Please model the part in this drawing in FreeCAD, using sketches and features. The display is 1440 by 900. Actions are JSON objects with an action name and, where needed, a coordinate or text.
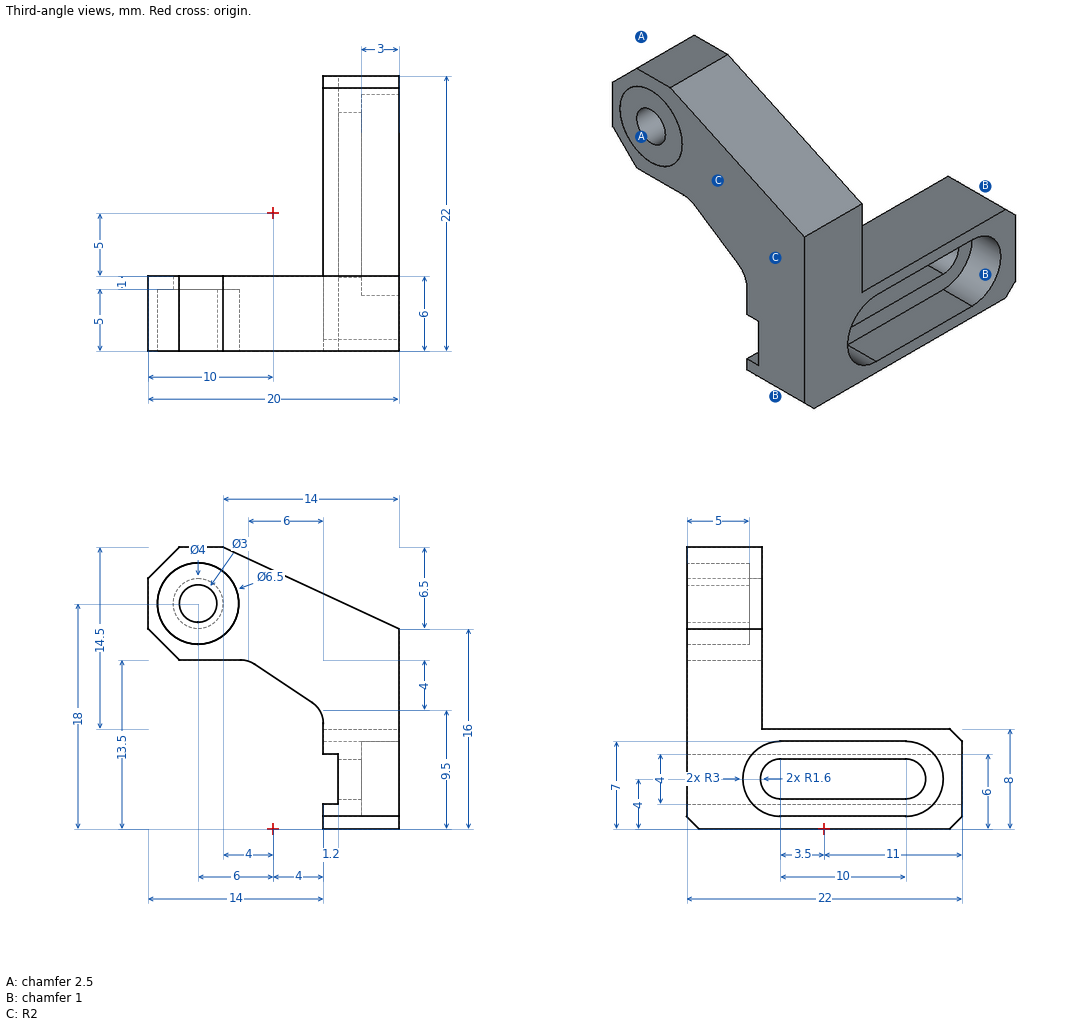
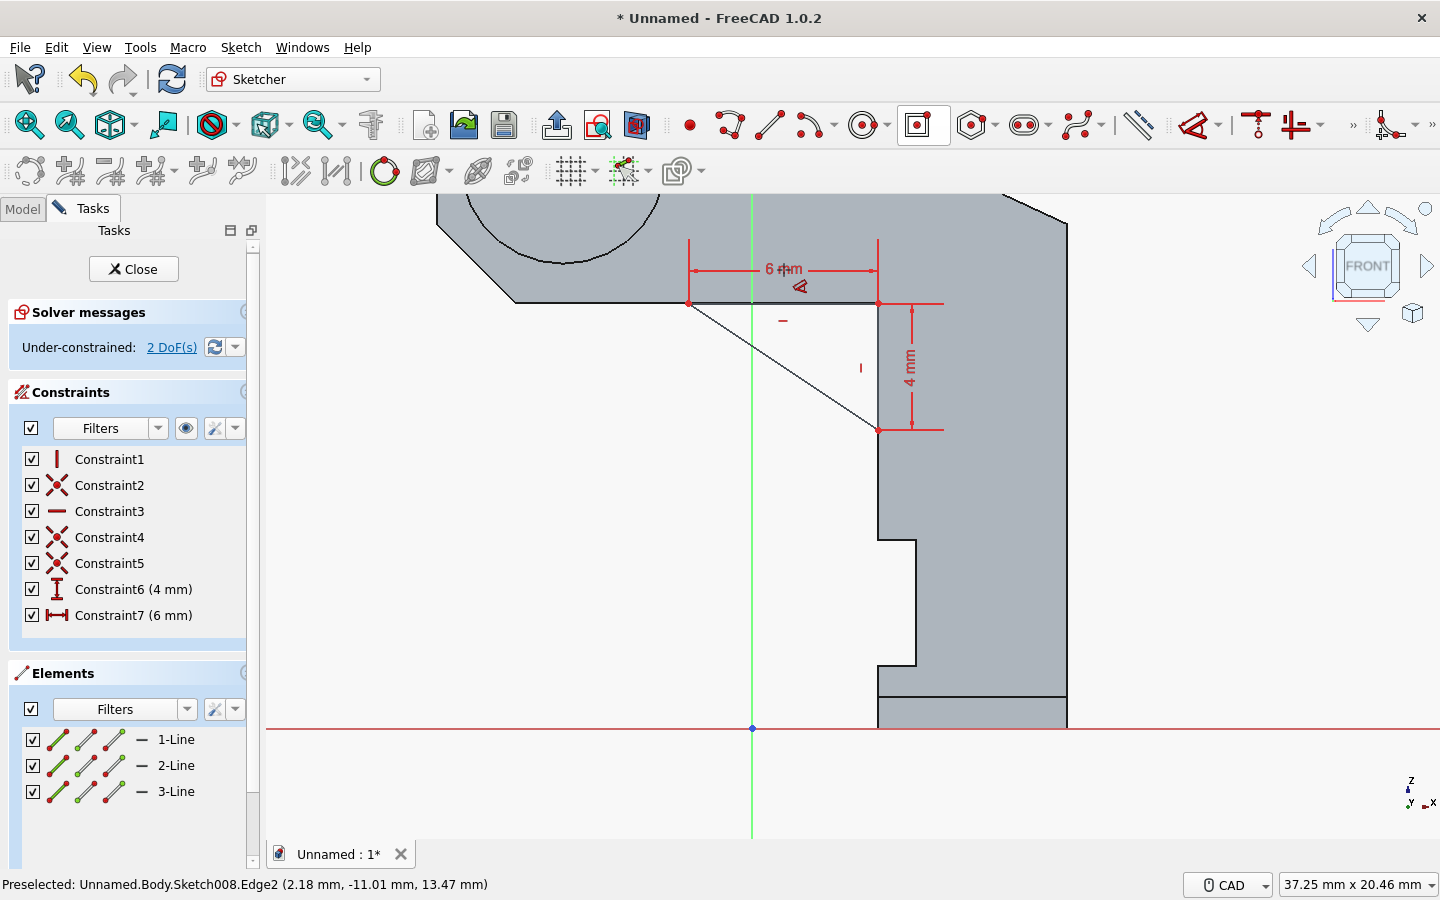
{"action": "left_click", "coordinate": [878, 430]}
{"action": "left_click", "coordinate": [815, 763]}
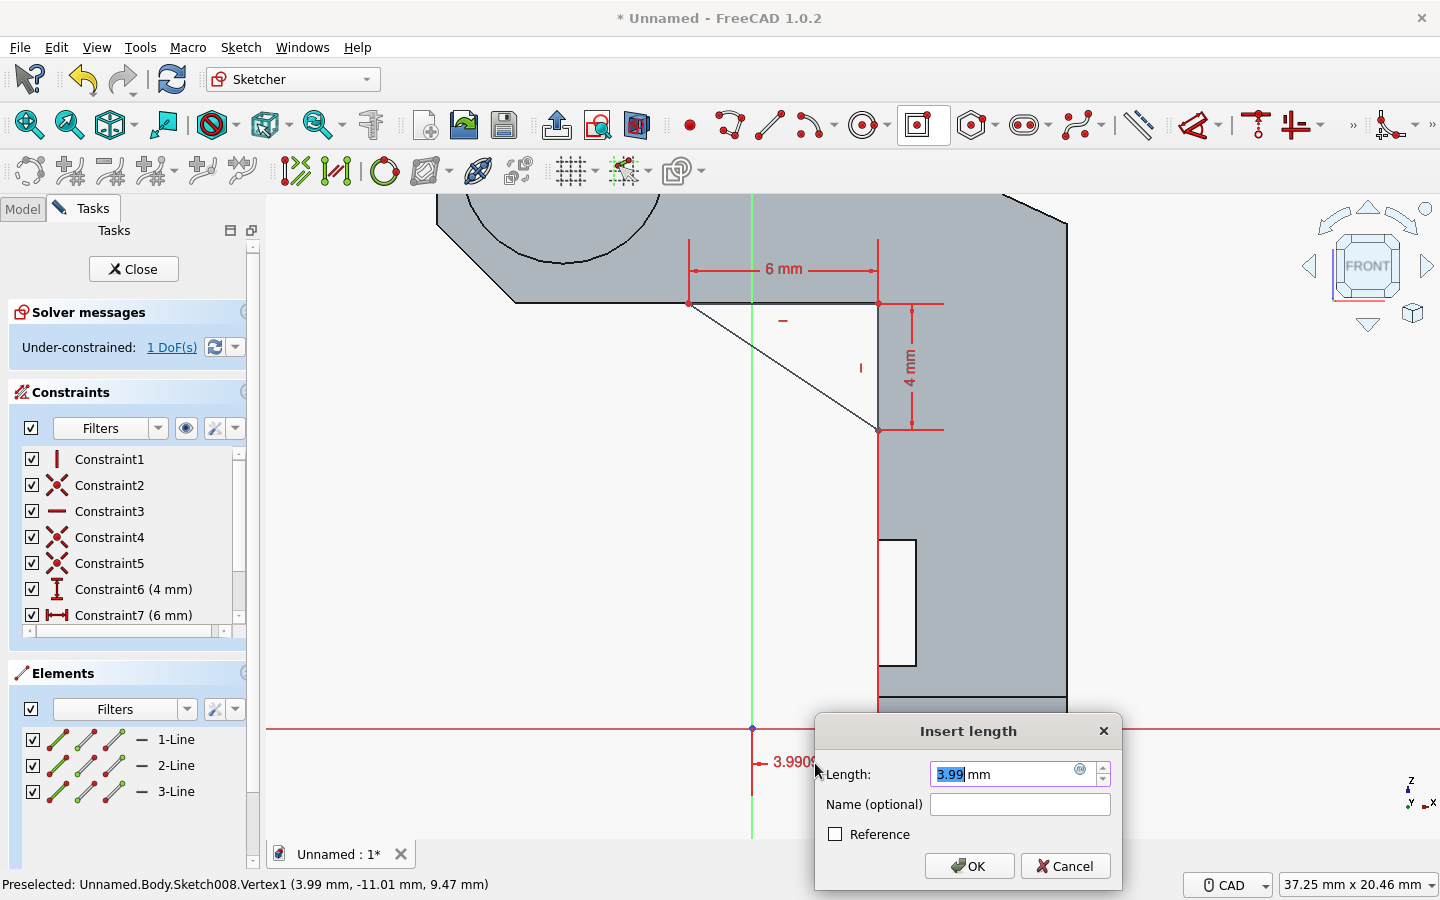
{"action": "type", "text": "4"}
{"action": "key", "text": "Return"}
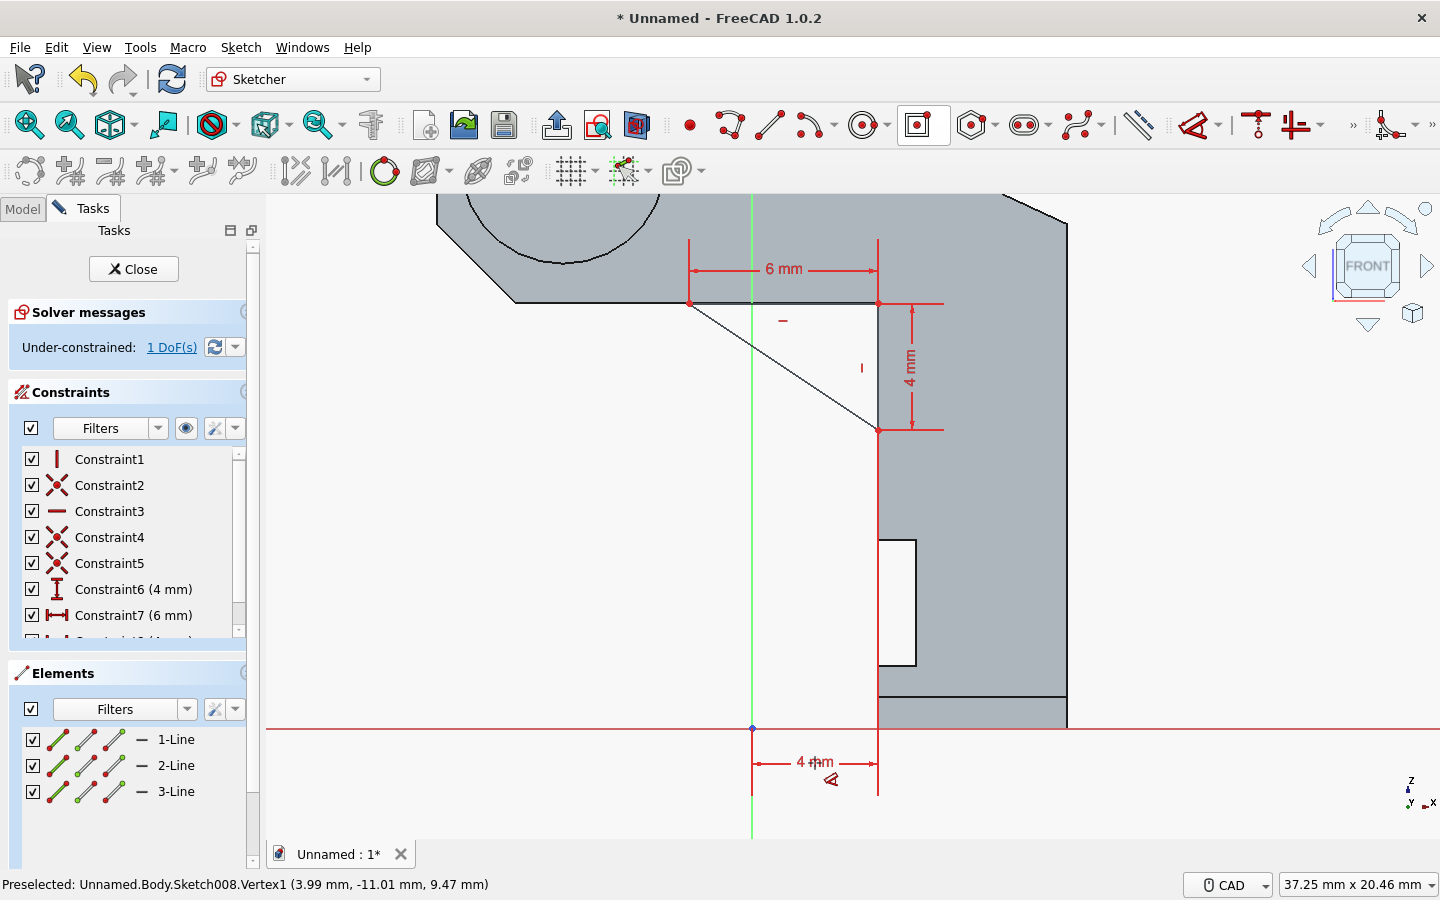
{"action": "left_click", "coordinate": [878, 430]}
{"action": "left_click", "coordinate": [912, 579]}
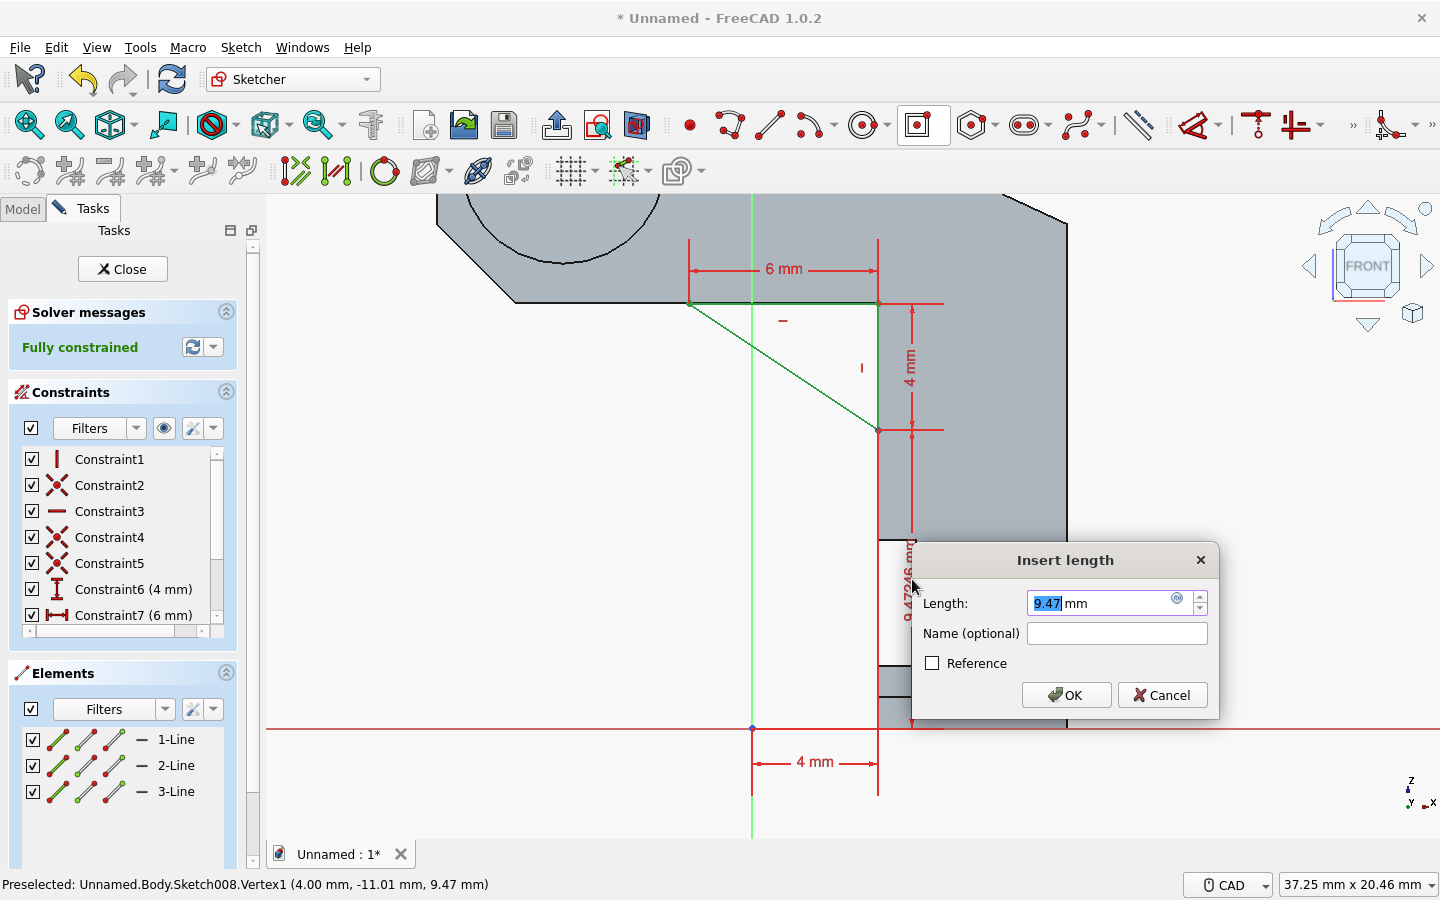
{"action": "type", "text": "9.5"}
{"action": "key", "text": "Return"}
{"action": "key", "text": "Escape"}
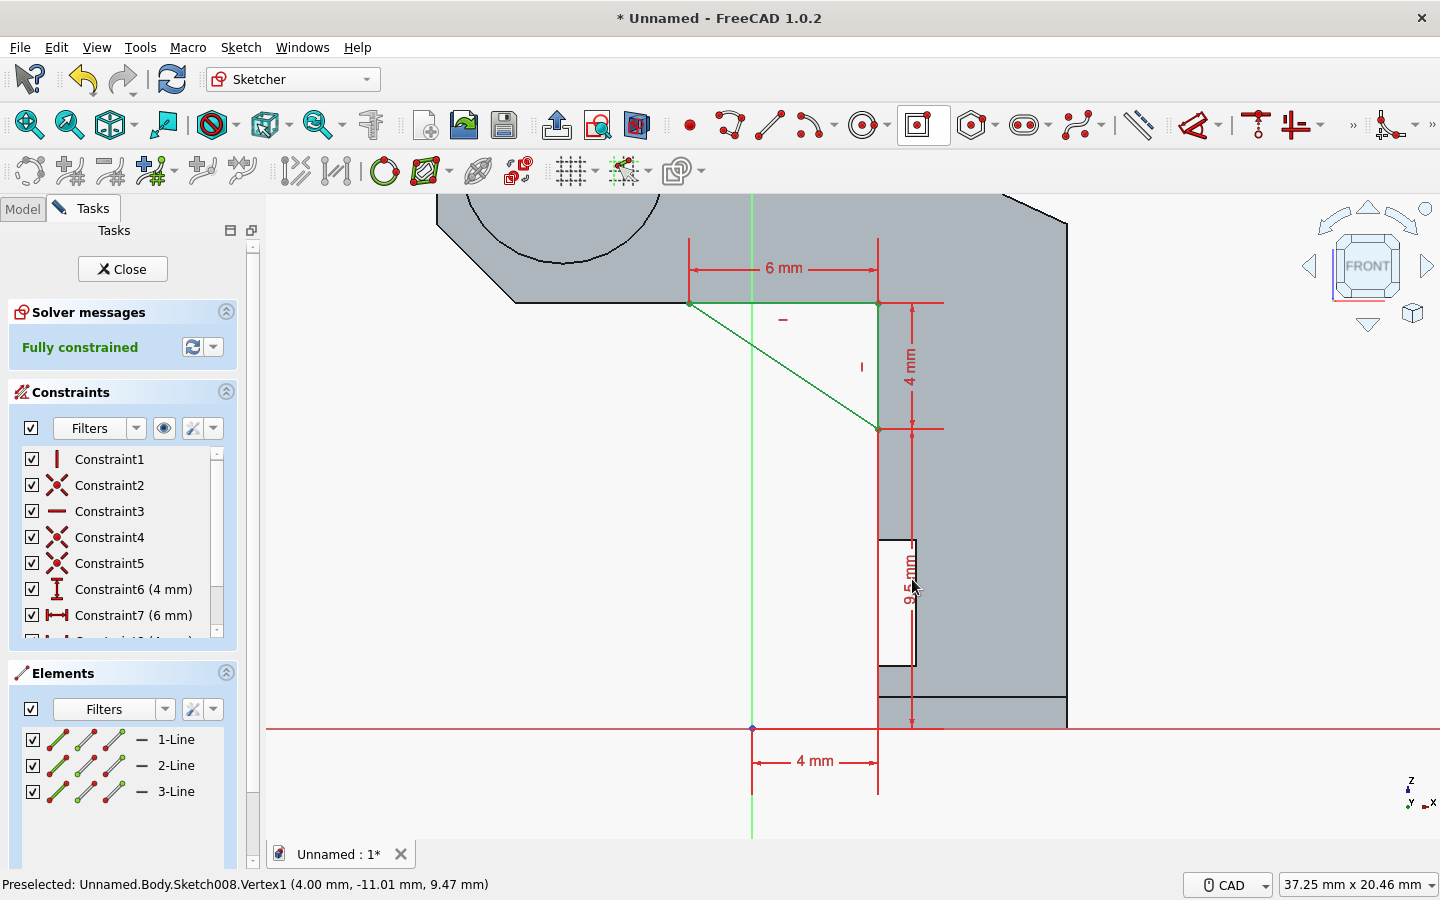
{"action": "left_click", "coordinate": [123, 269]}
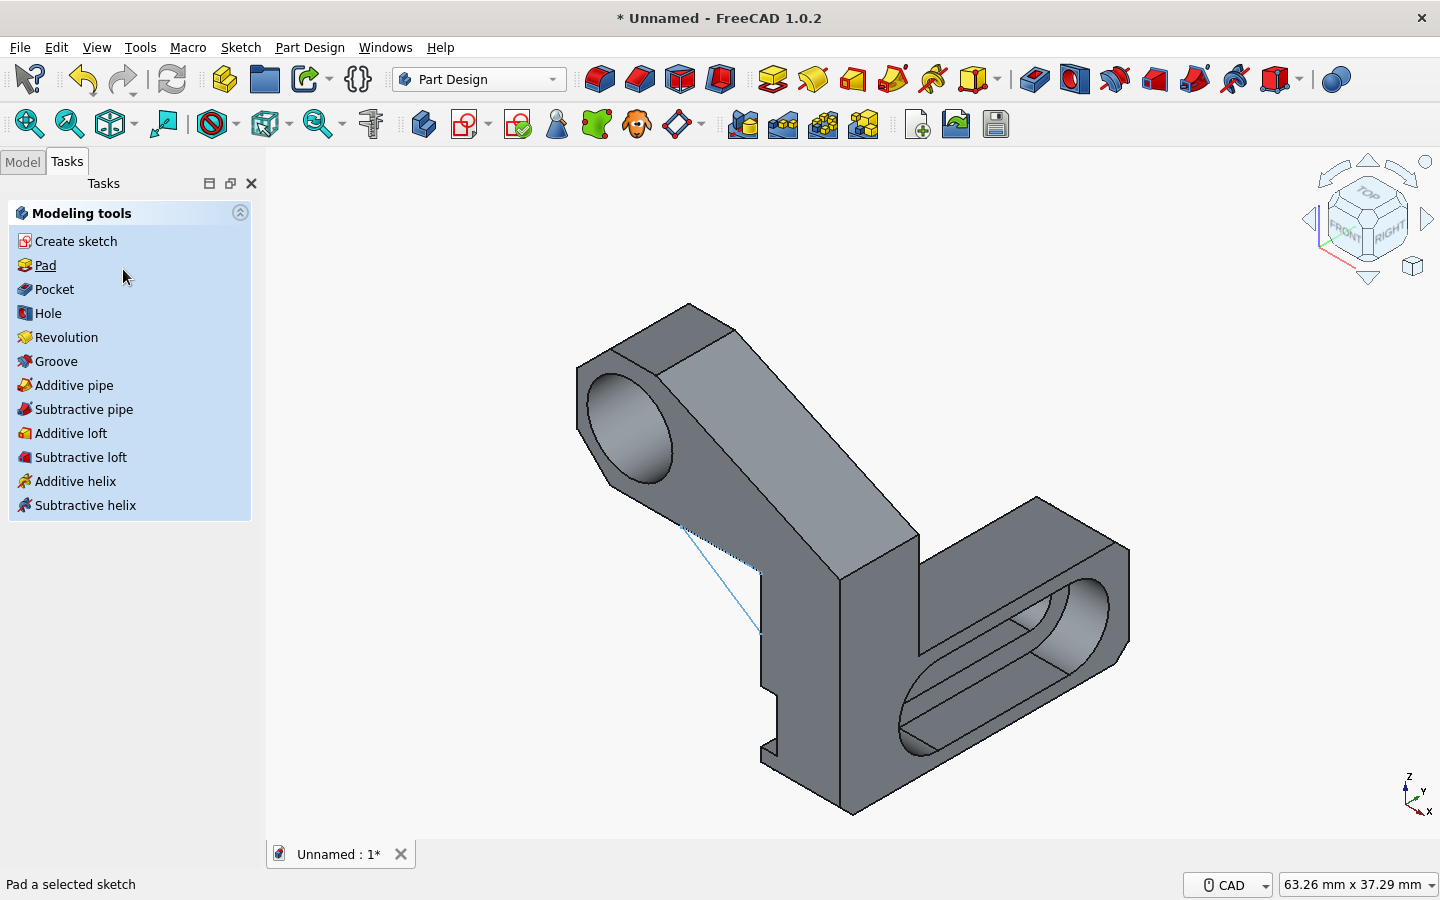
{"action": "left_click", "coordinate": [774, 80]}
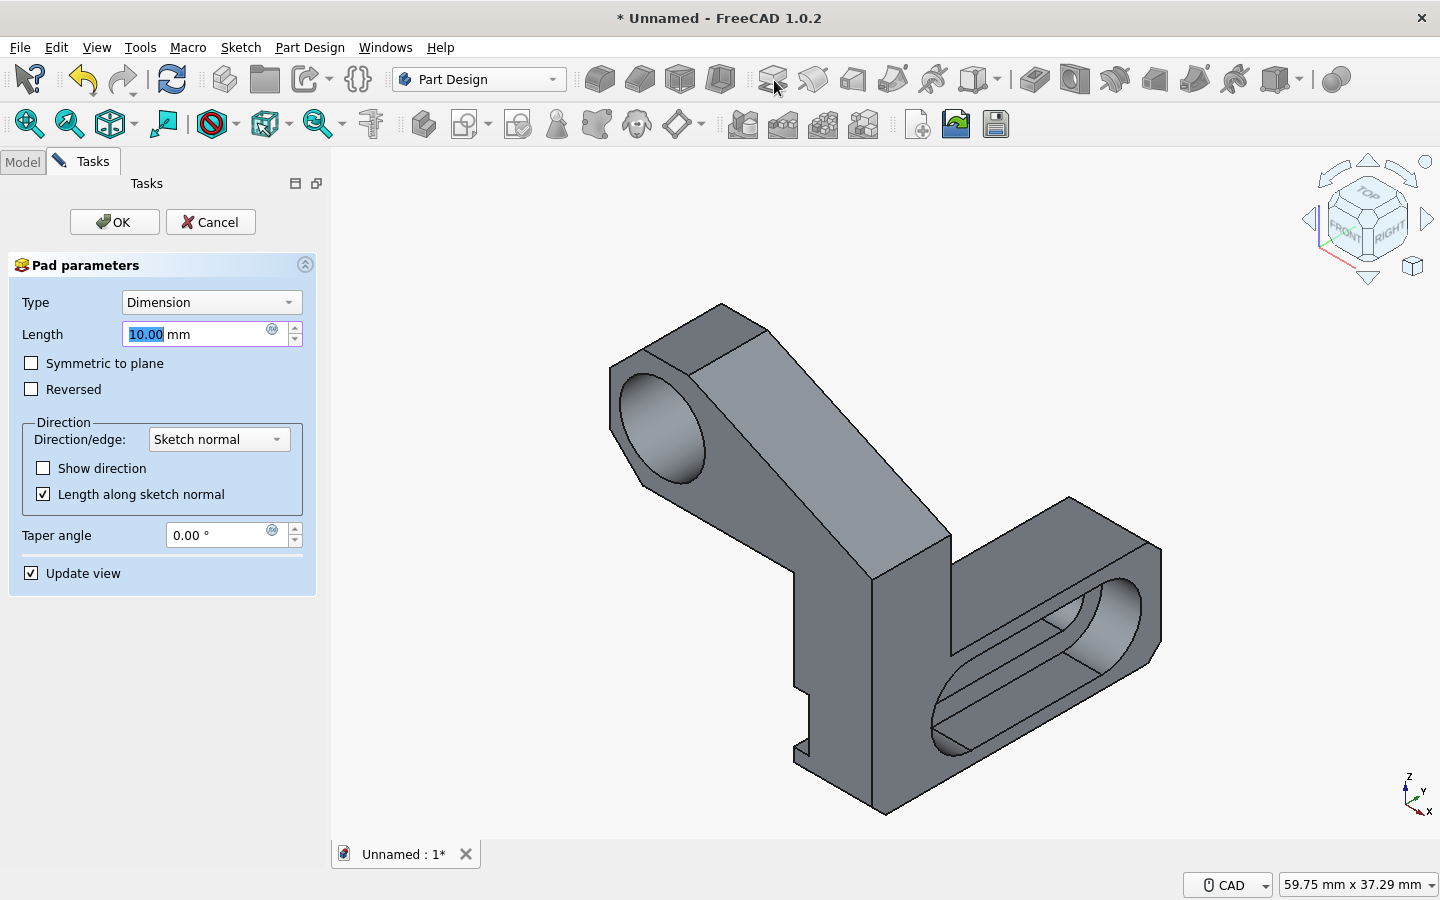
{"action": "type", "text": "6"}
{"action": "key", "text": "Tab"}